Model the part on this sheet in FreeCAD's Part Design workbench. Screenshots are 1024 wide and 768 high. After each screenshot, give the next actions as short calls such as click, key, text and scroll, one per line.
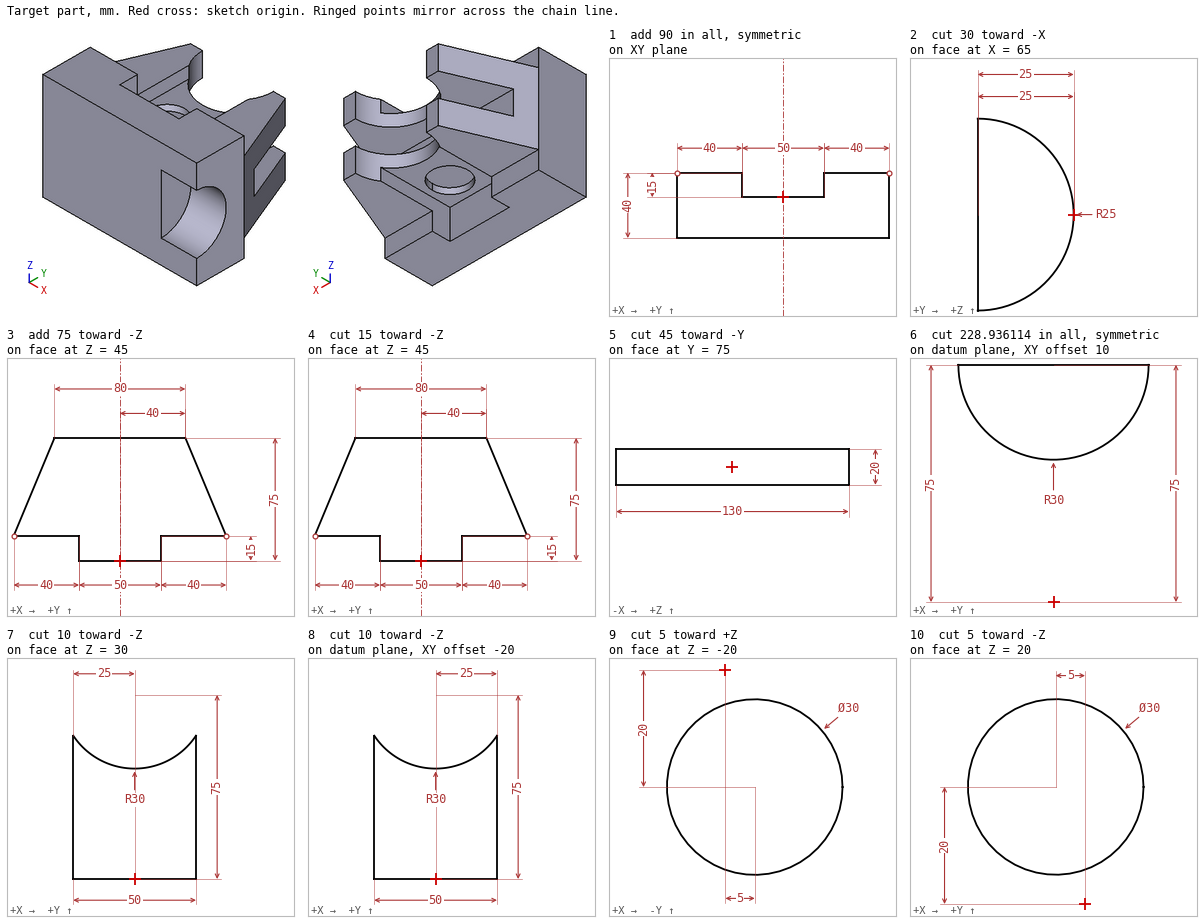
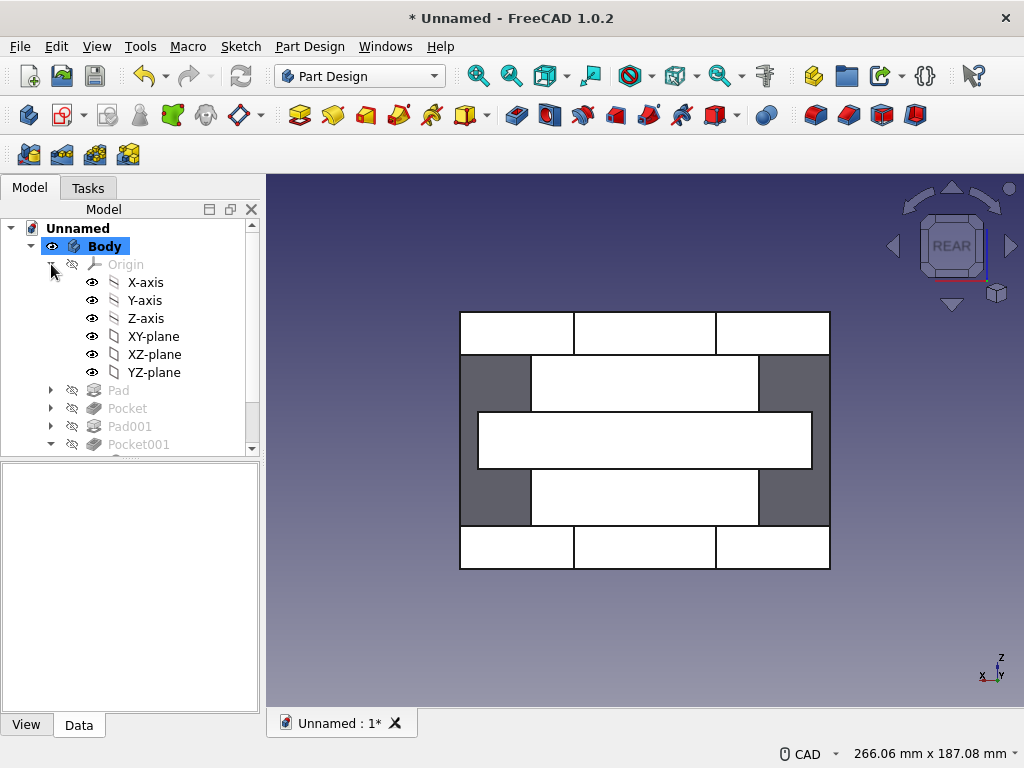
click(137, 336)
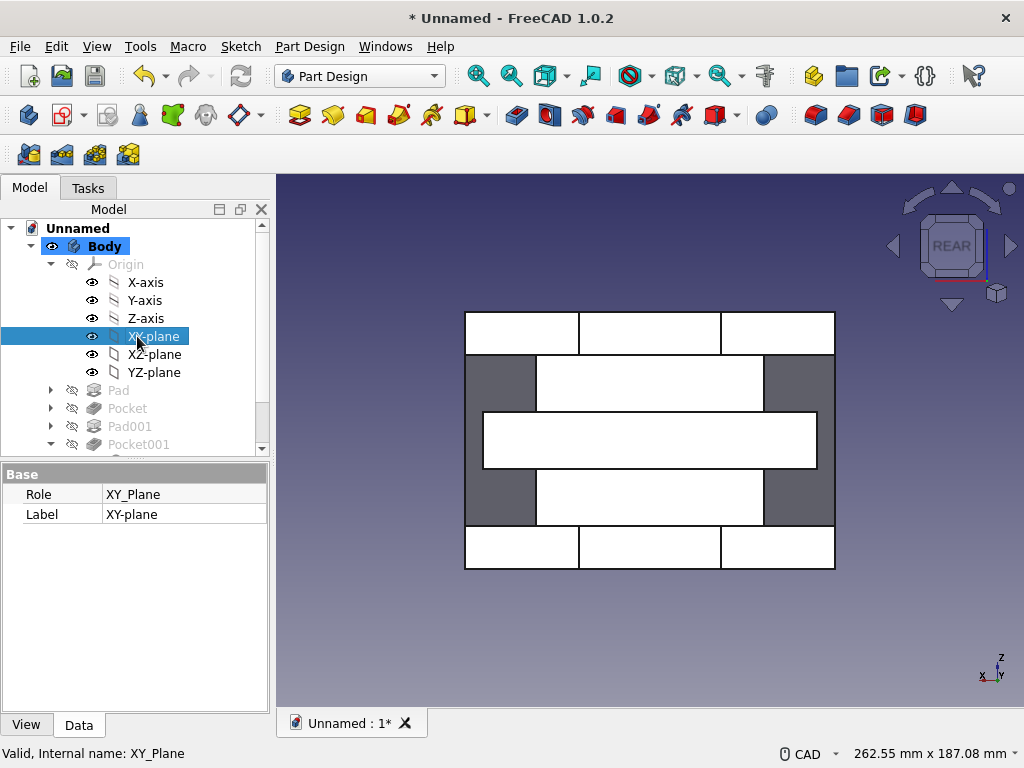
click(238, 116)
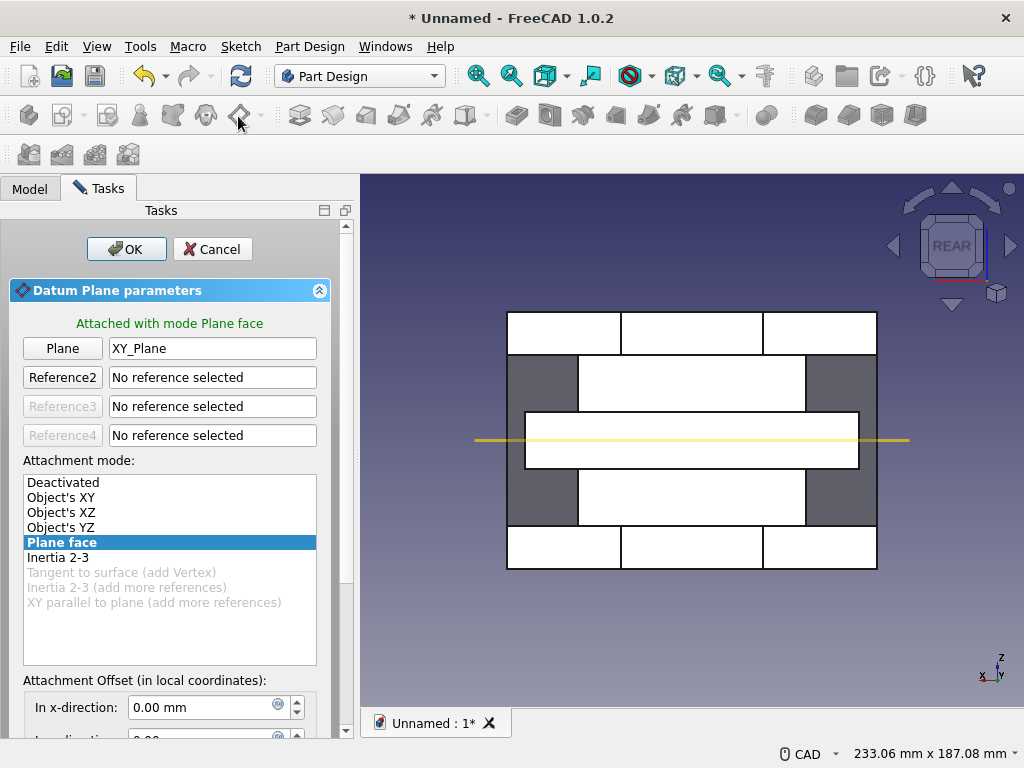
scroll(346, 479, down, 2)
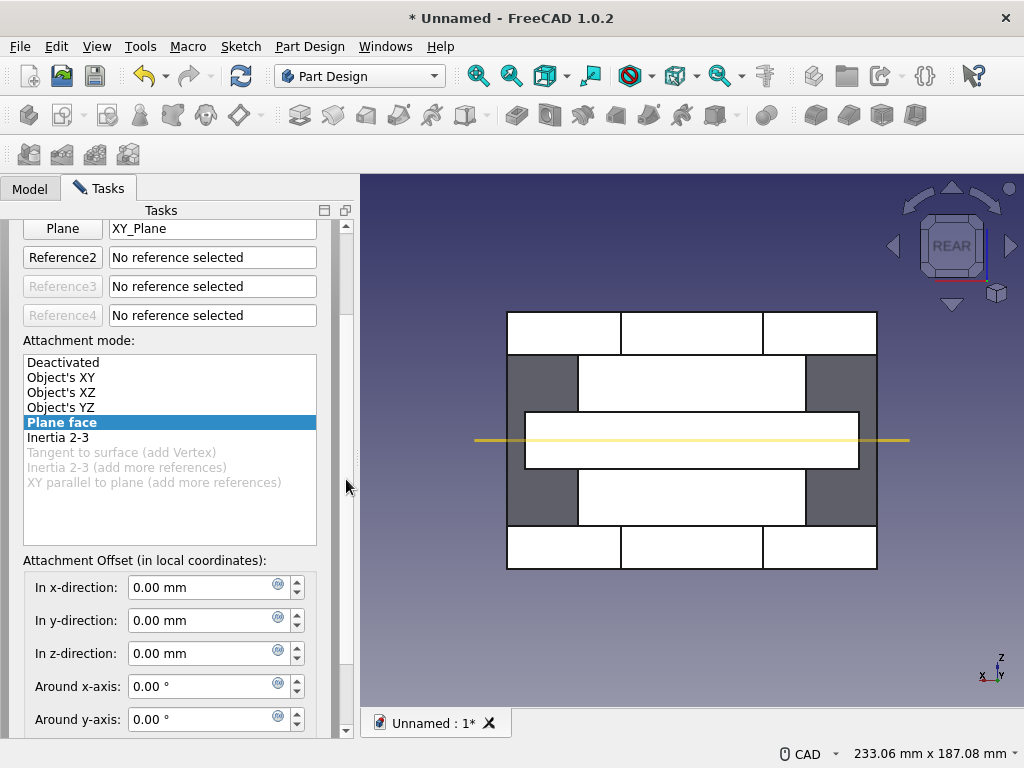
triple_click(210, 654)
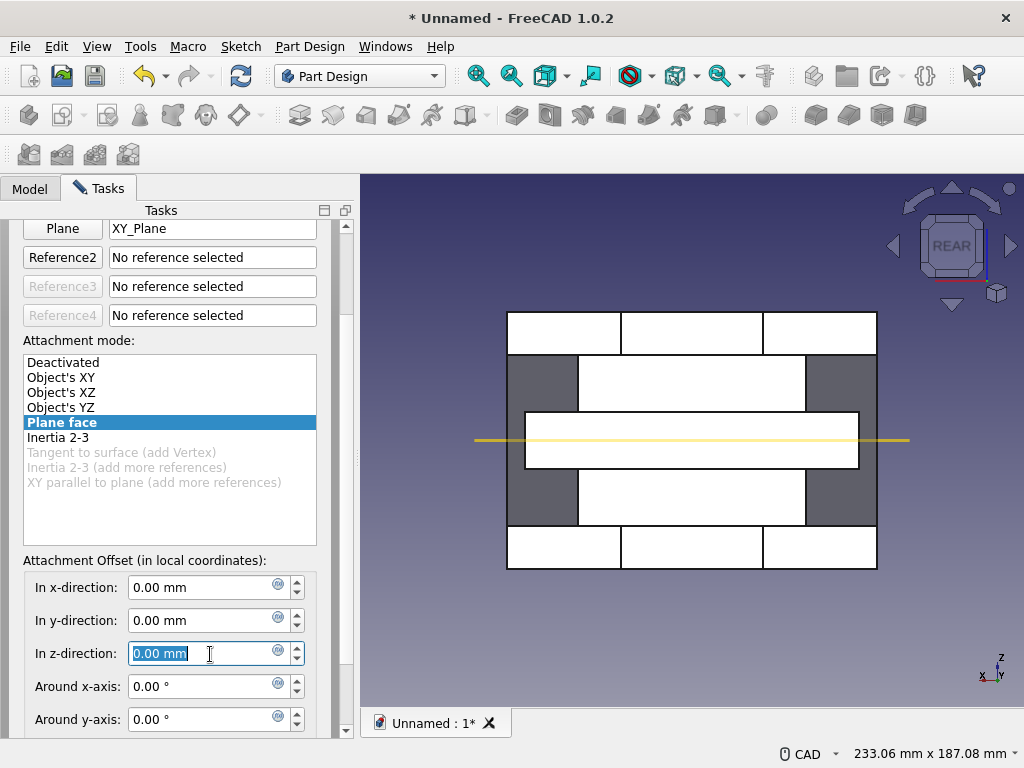
text(10)
key(Tab)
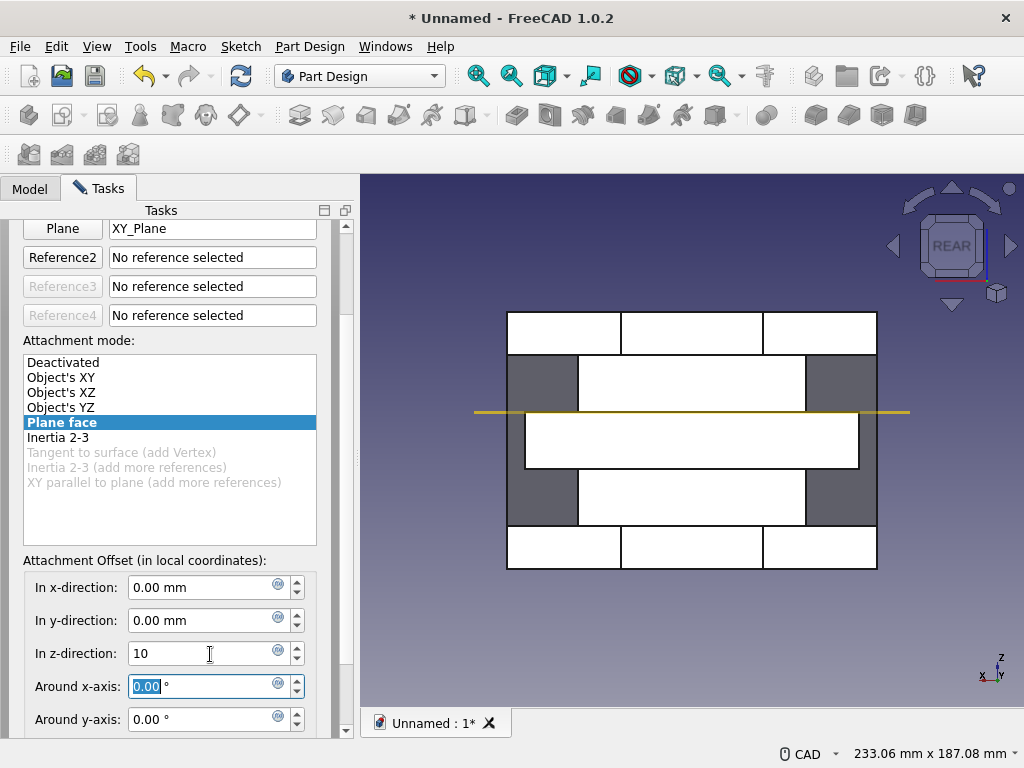
scroll(346, 479, up, 3)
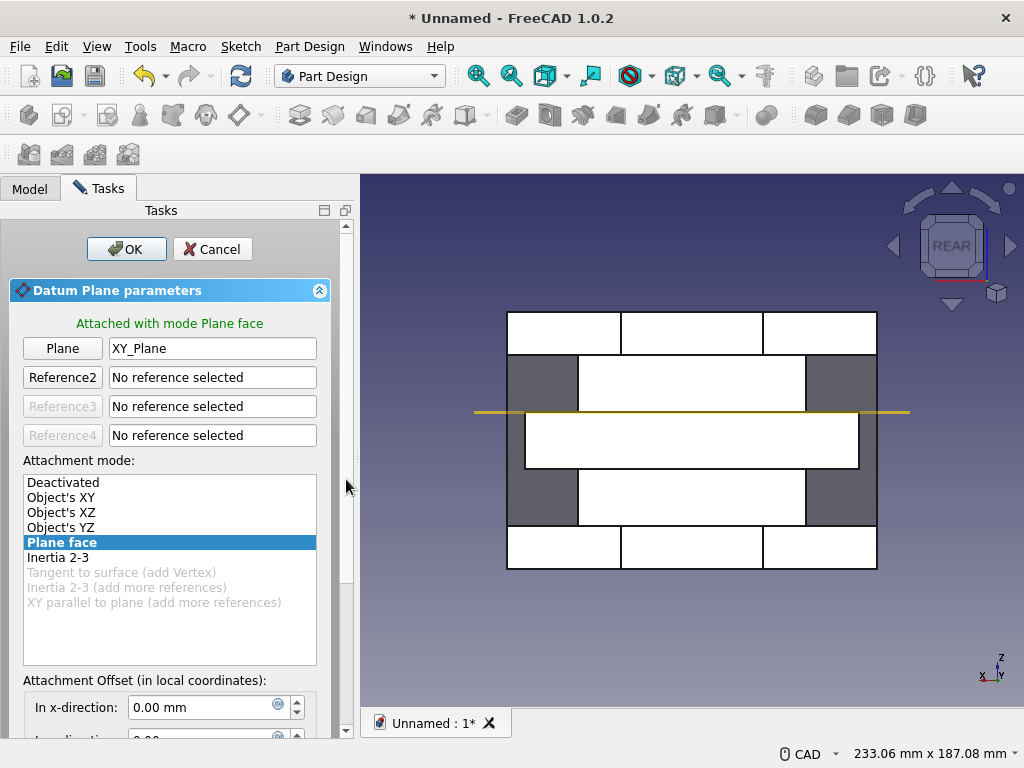
click(127, 249)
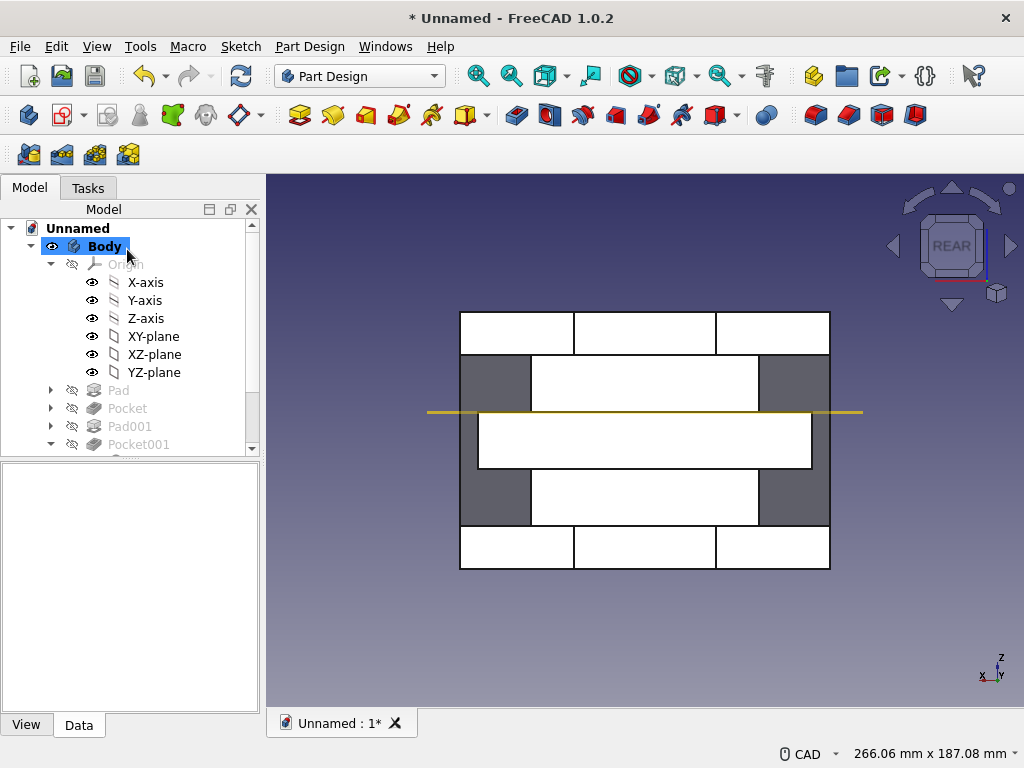
scroll(101, 332, down, 3)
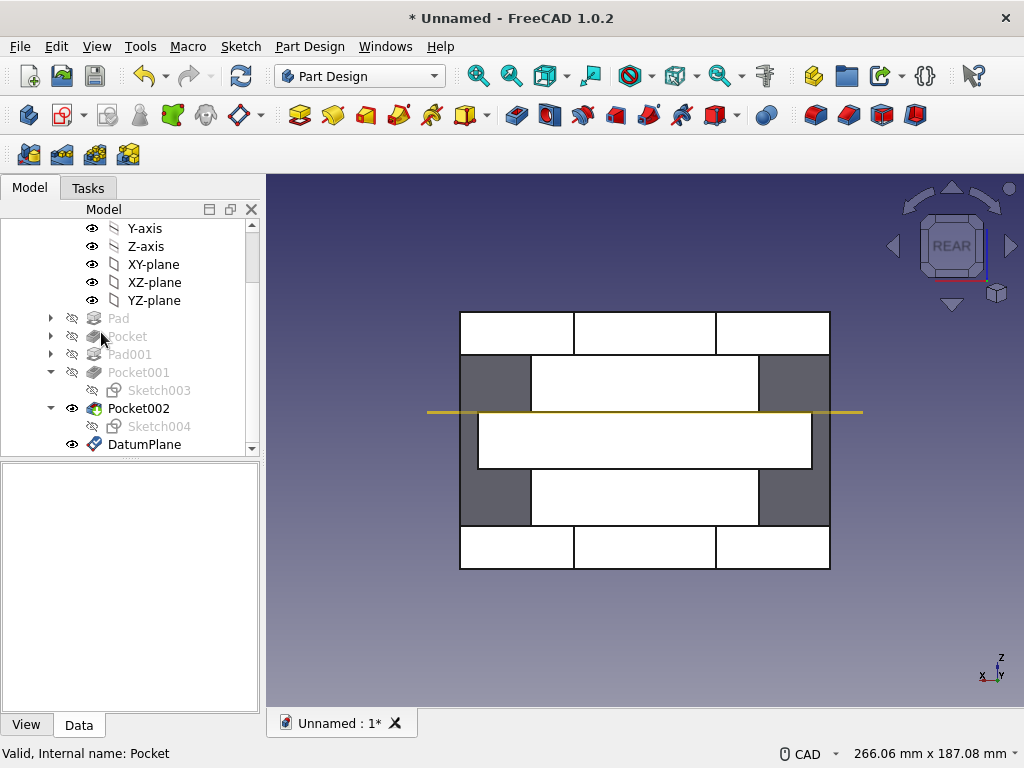
click(117, 444)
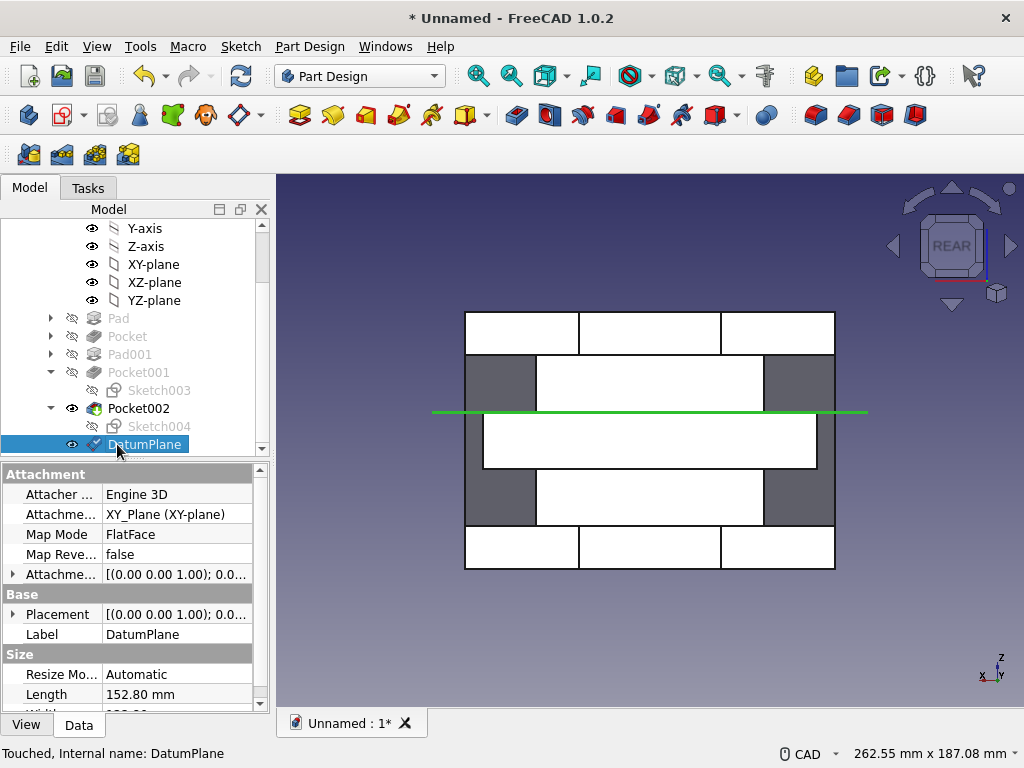
click(62, 116)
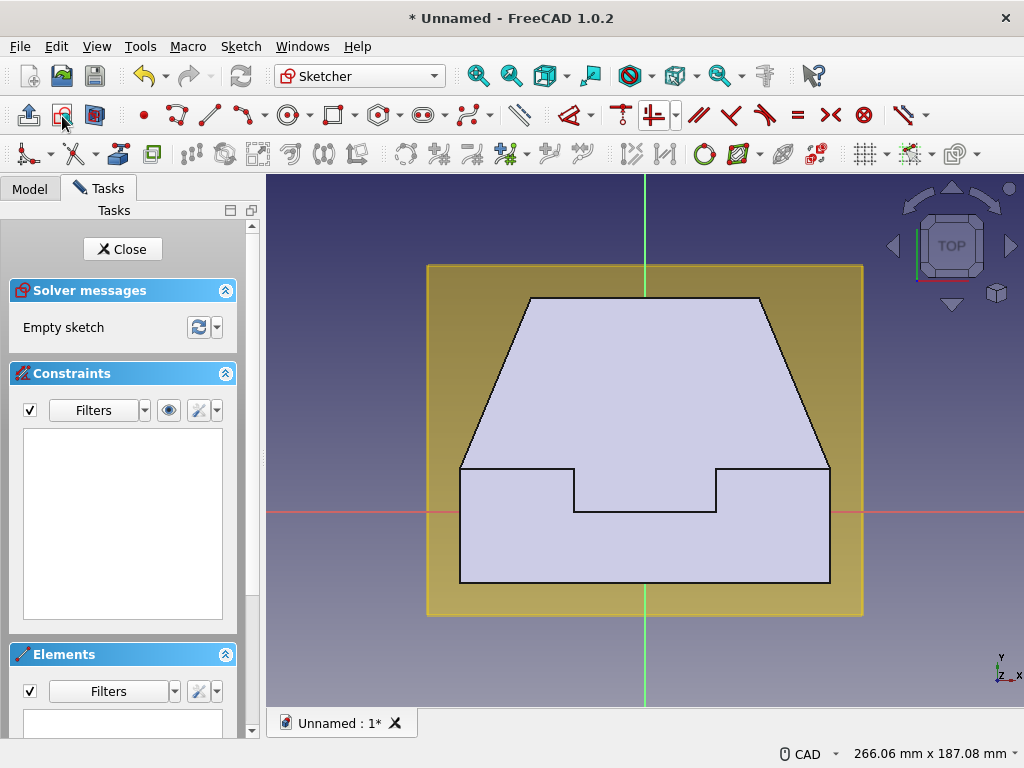
key(q)
key(s)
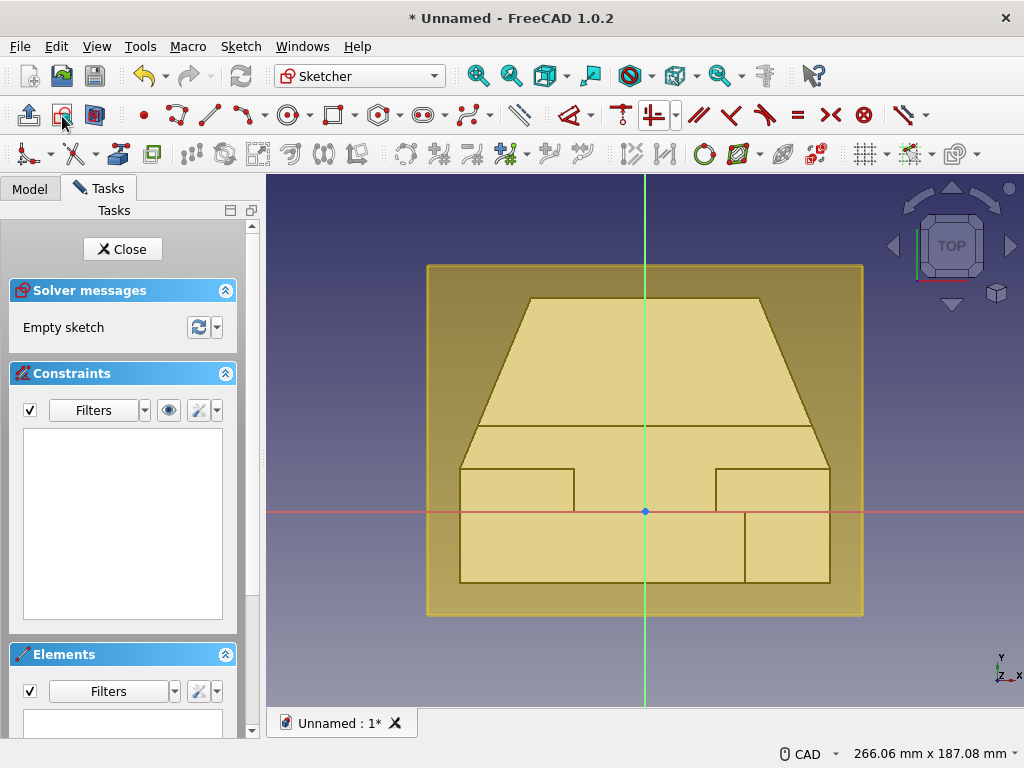
scroll(784, 332, up, 2)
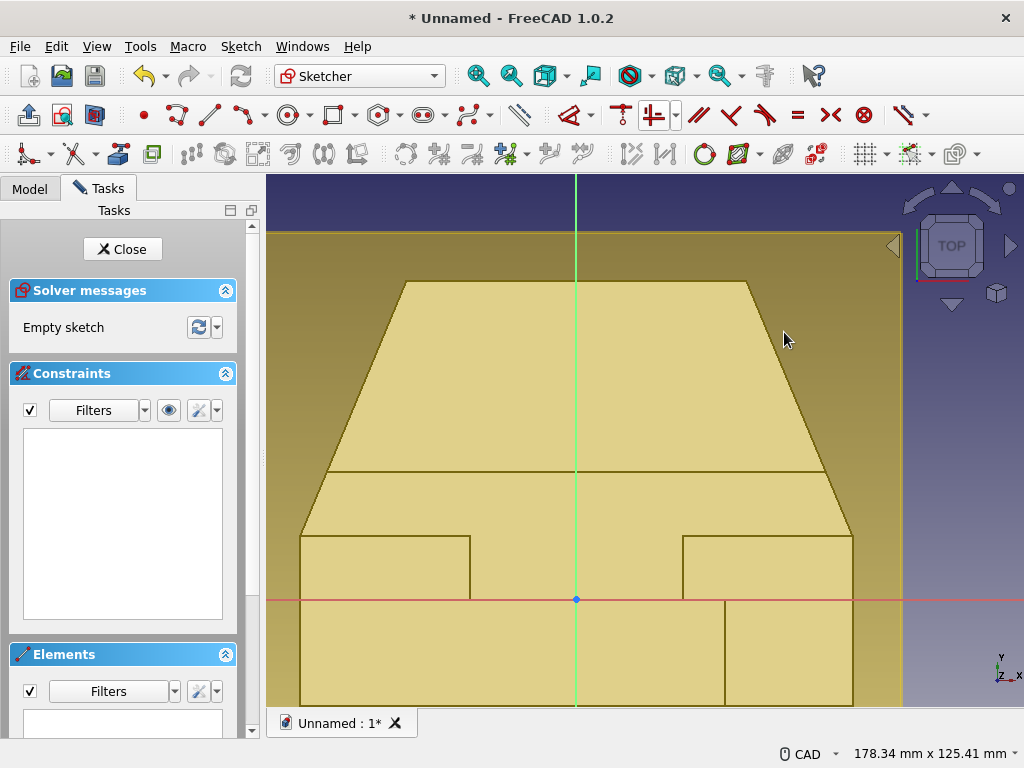
click(210, 116)